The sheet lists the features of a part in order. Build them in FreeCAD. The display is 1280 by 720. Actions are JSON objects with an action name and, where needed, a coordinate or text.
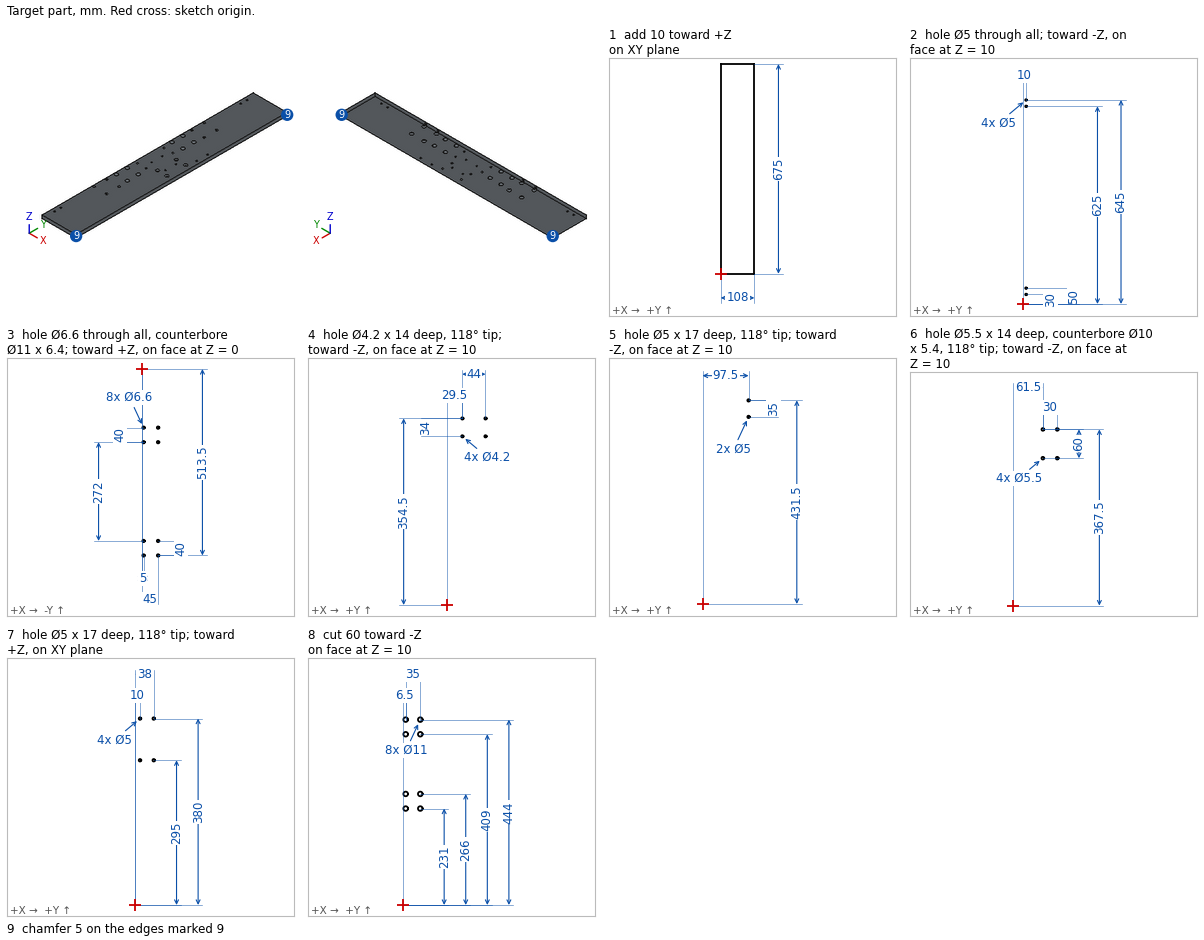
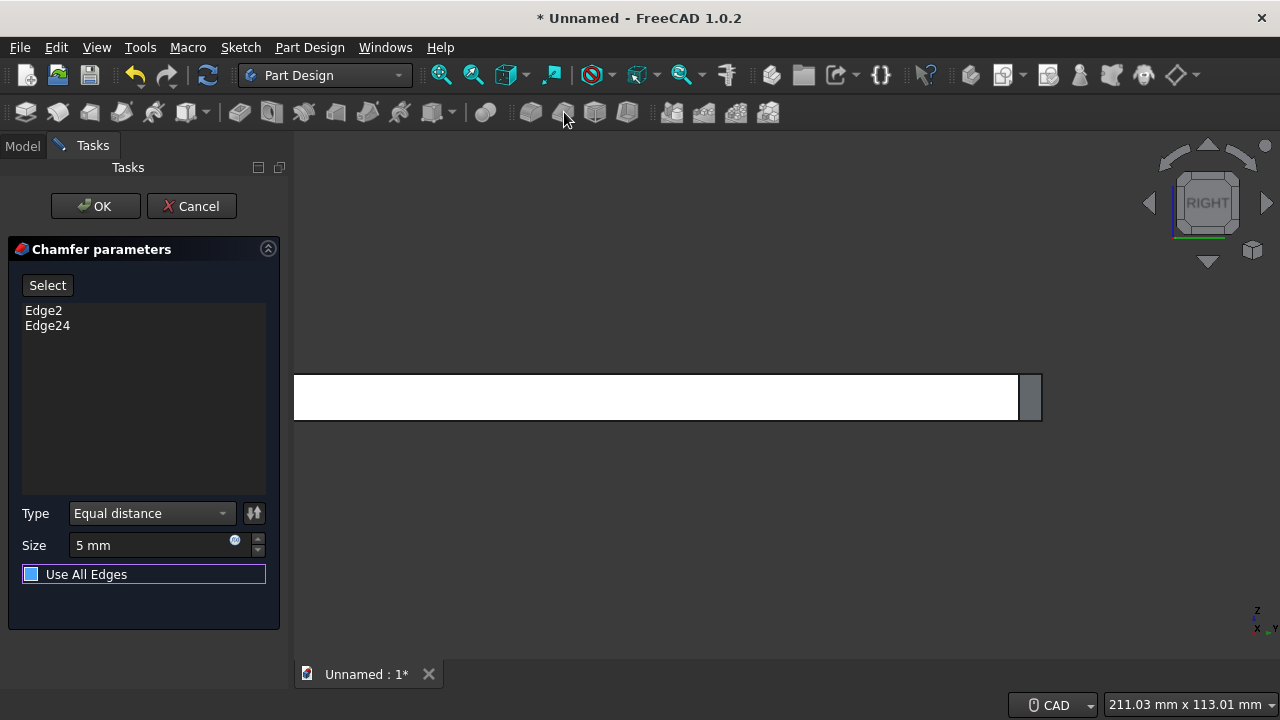
{"action": "left_click", "coordinate": [96, 206]}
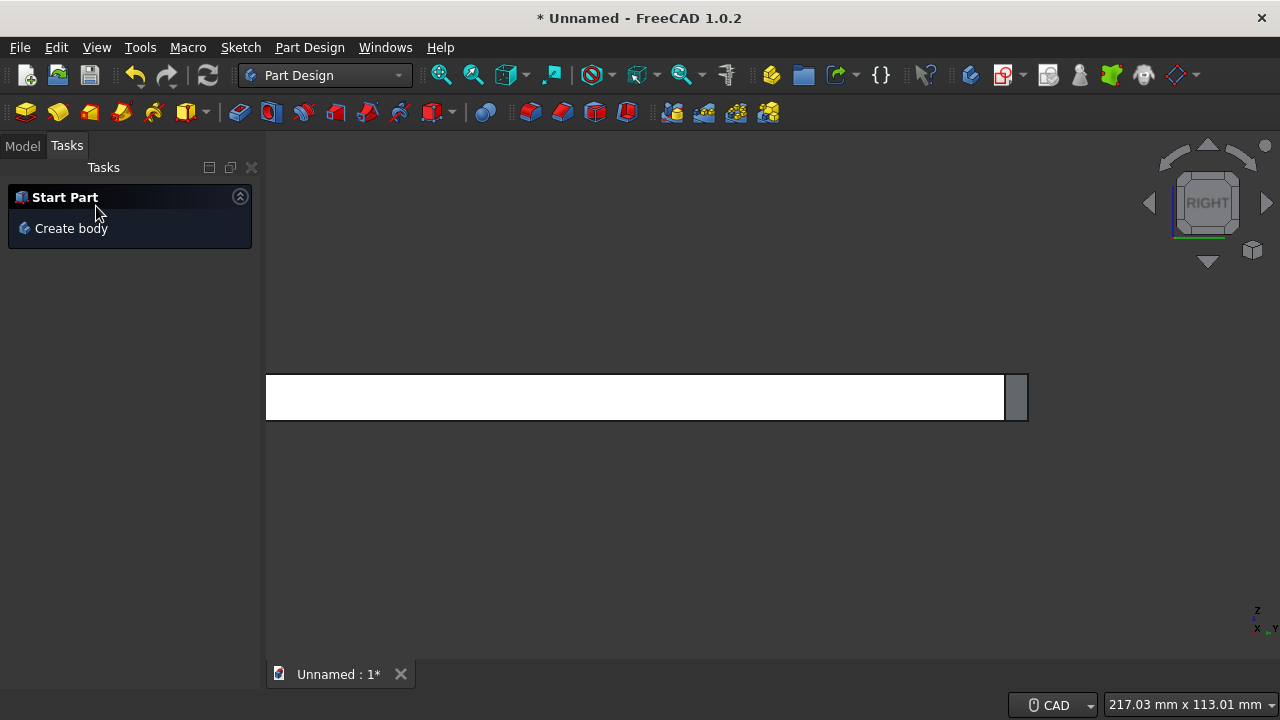
{"action": "key", "text": "0"}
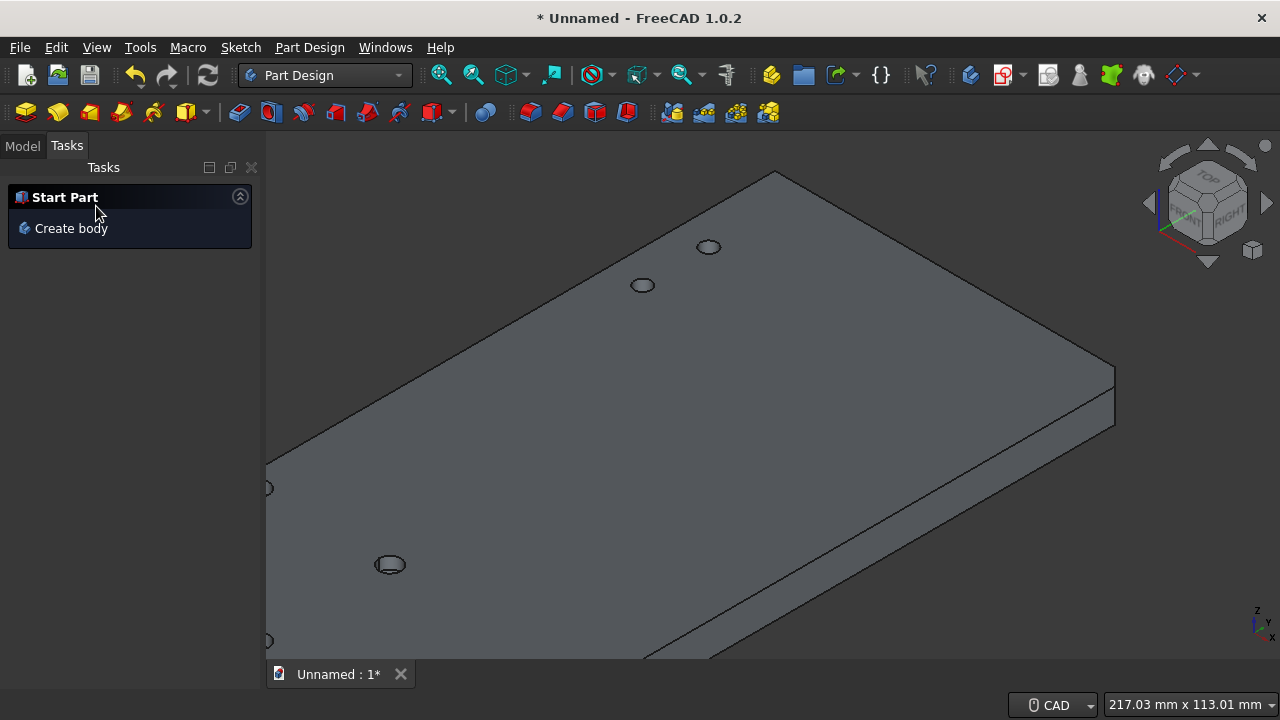
{"action": "key", "text": "v f"}